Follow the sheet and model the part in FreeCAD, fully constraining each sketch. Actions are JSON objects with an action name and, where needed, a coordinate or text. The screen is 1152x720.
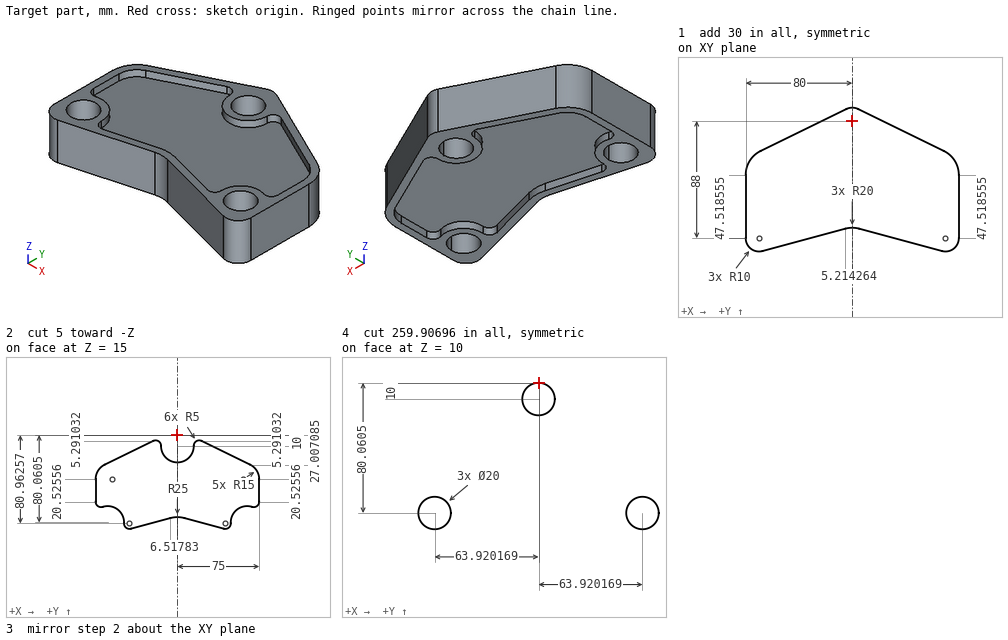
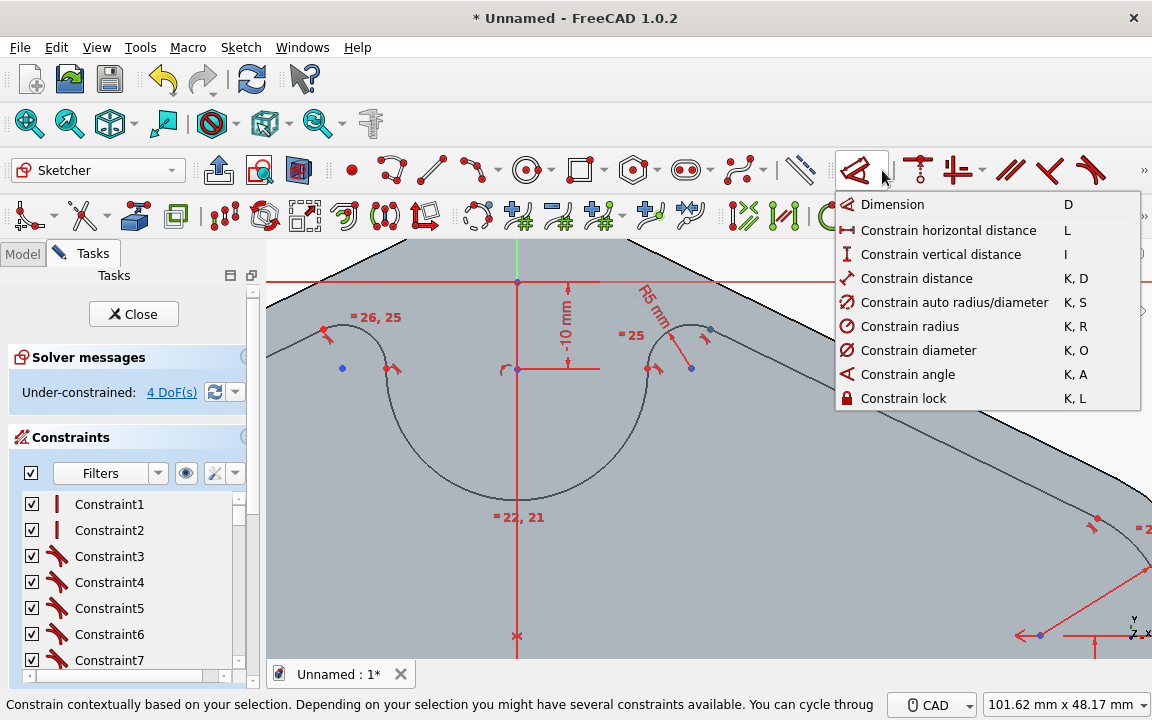
{"action": "left_click", "coordinate": [988, 254]}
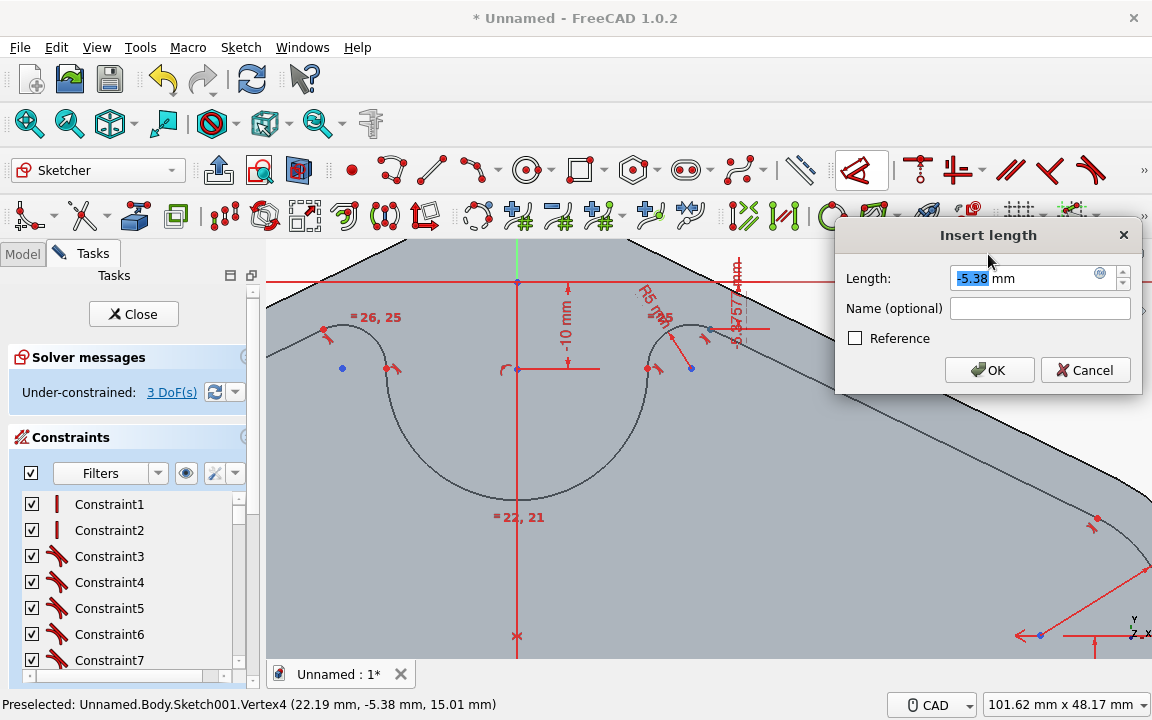
{"action": "type", "text": "-5.291032"}
{"action": "key", "text": "Return"}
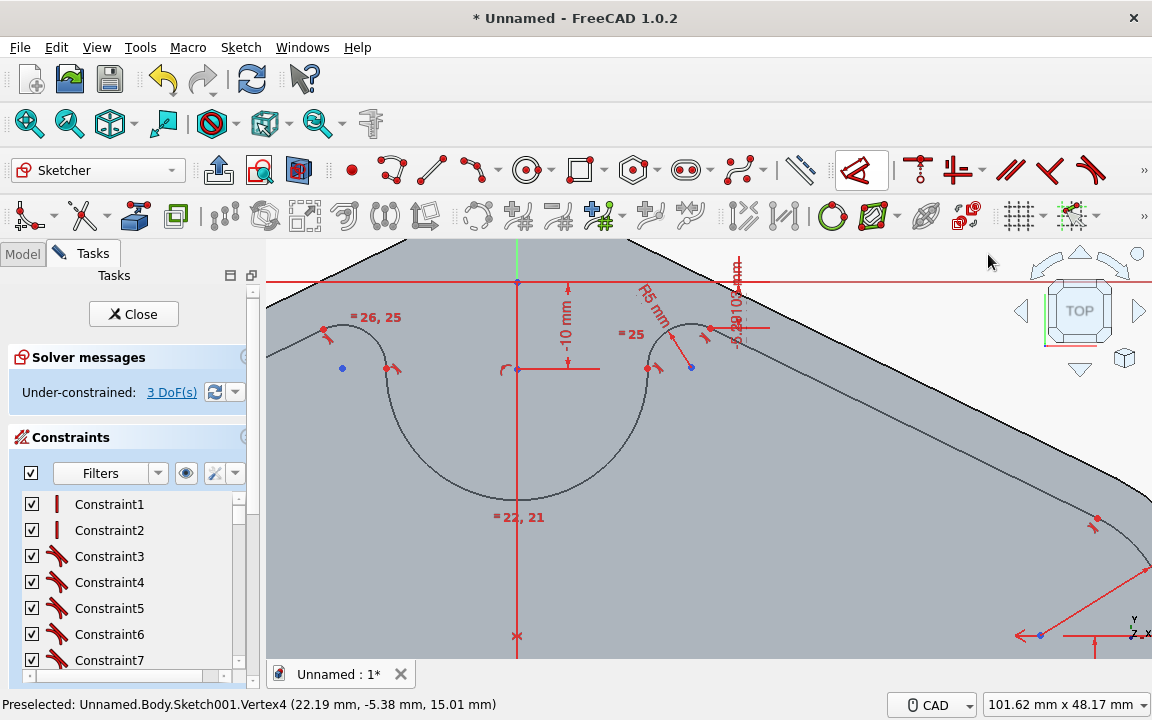
{"action": "left_click", "coordinate": [324, 329]}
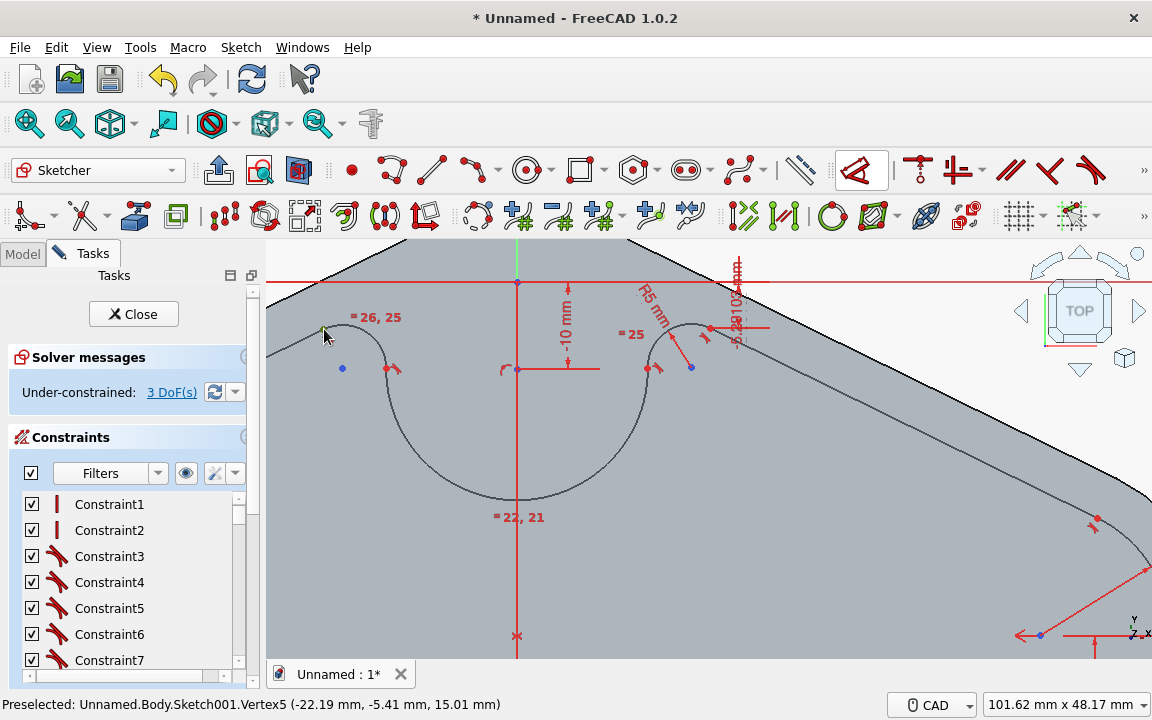
{"action": "key", "text": "i"}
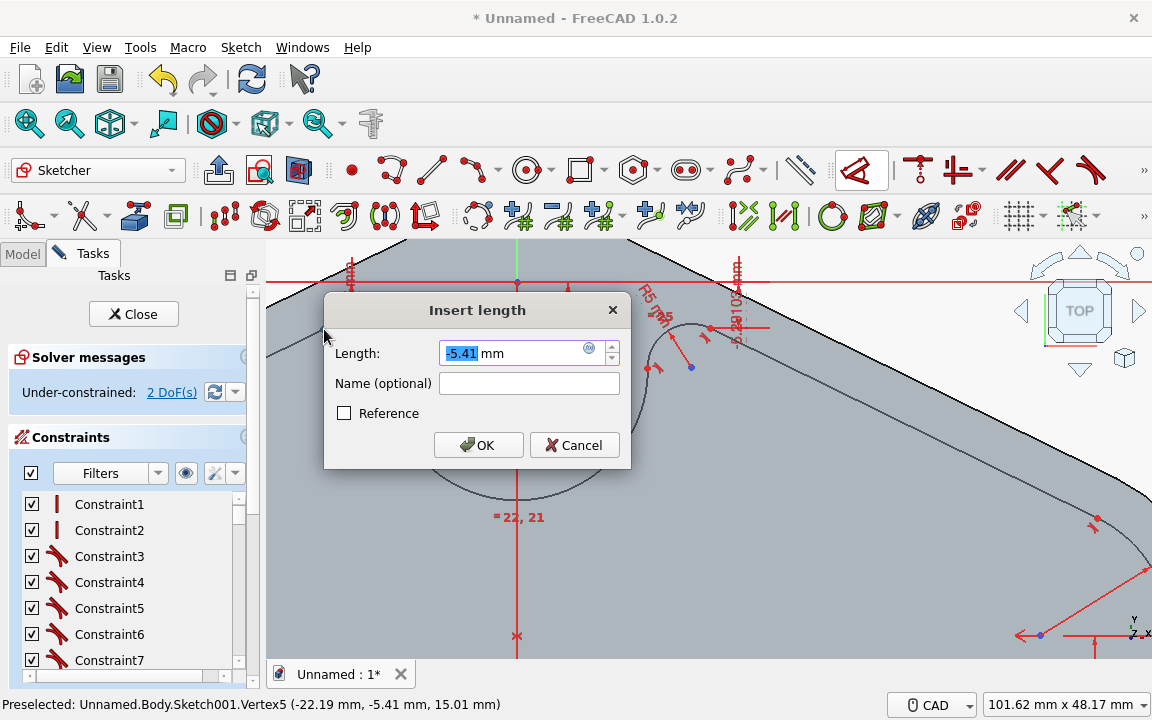
{"action": "type", "text": "-5.291032"}
{"action": "key", "text": "Return"}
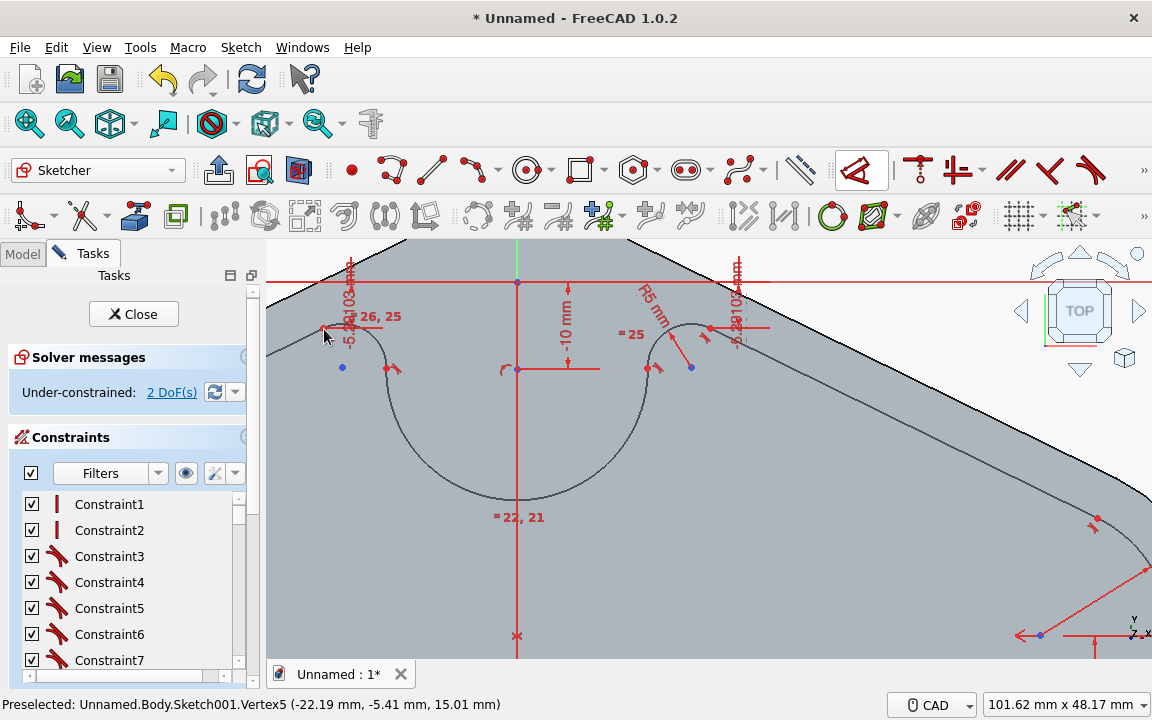
{"action": "scroll", "coordinate": [712, 328], "scroll_direction": "down", "scroll_amount": 5}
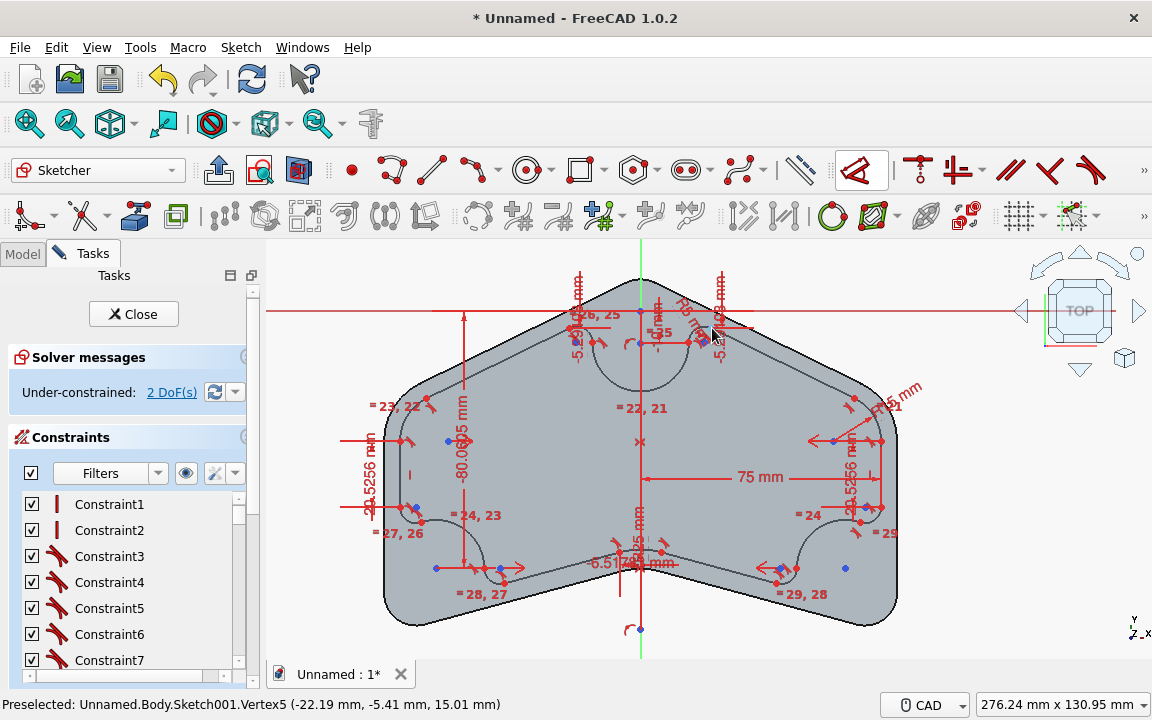
{"action": "left_click", "coordinate": [500, 568]}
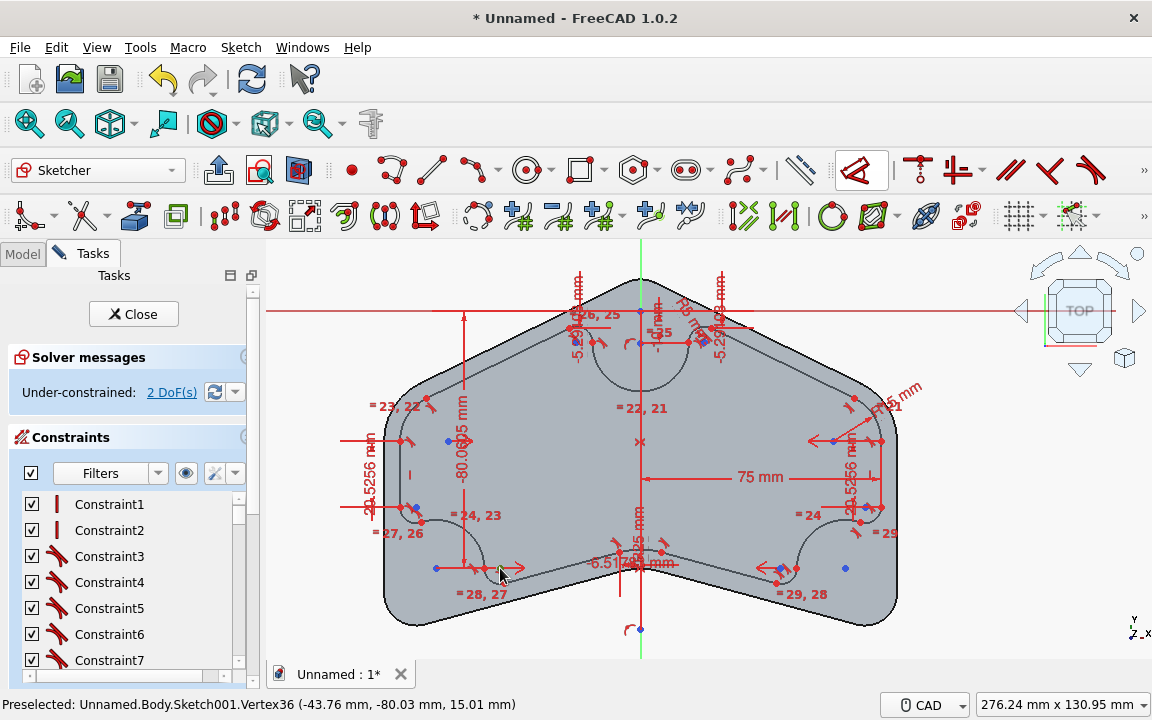
{"action": "key", "text": "i"}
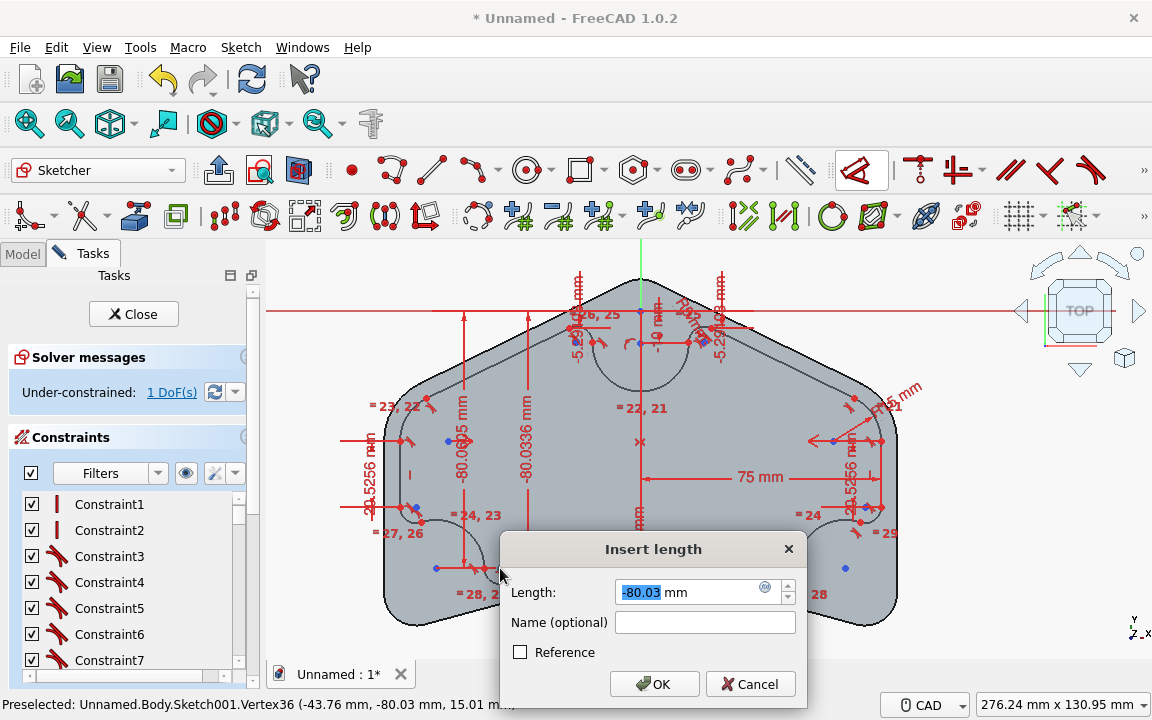
{"action": "type", "text": "-80.96257"}
{"action": "key", "text": "Return"}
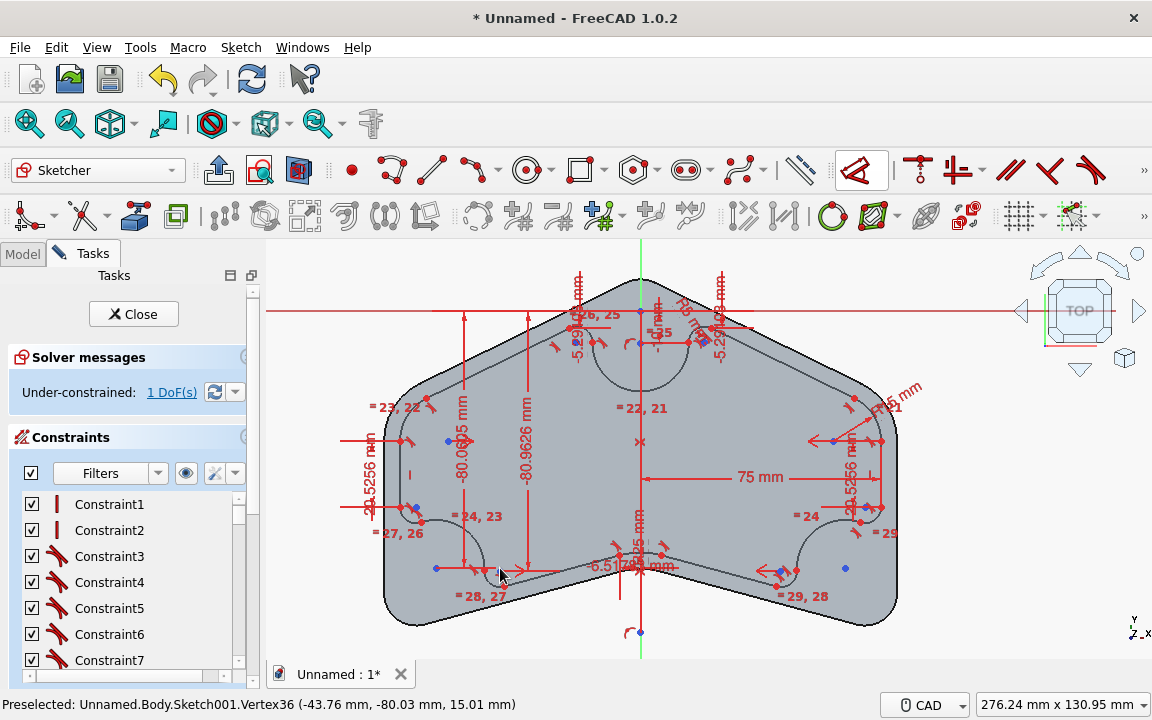
{"action": "left_click", "coordinate": [854, 398]}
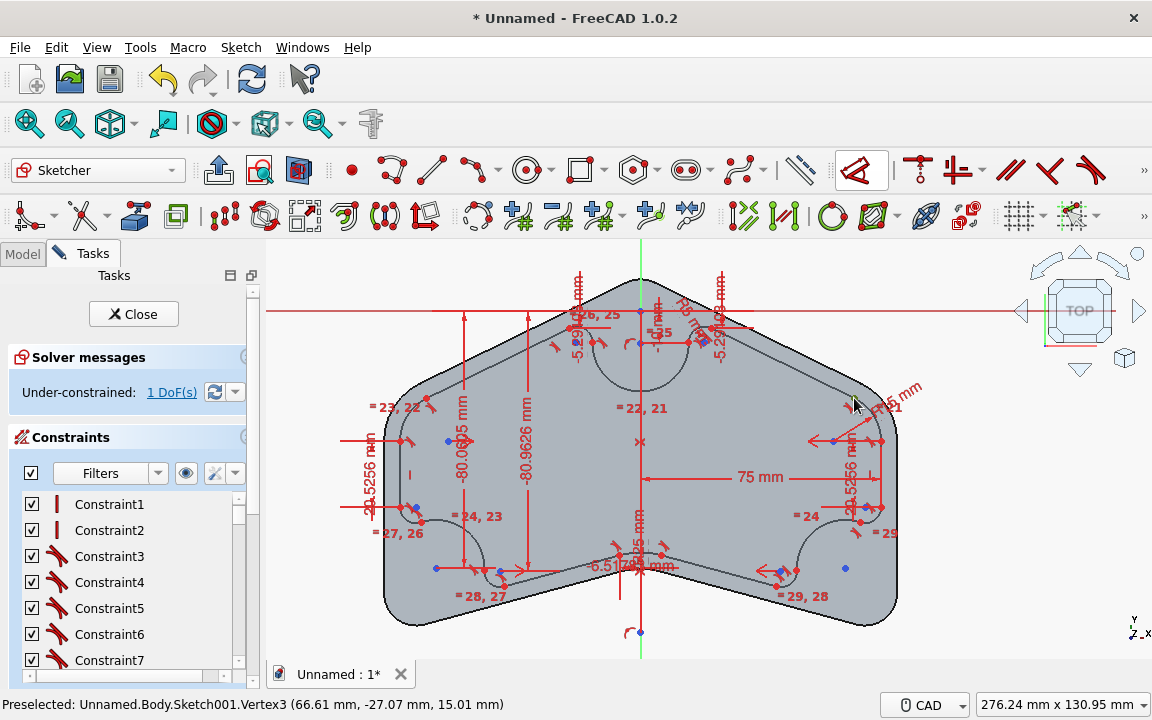
{"action": "key", "text": "i"}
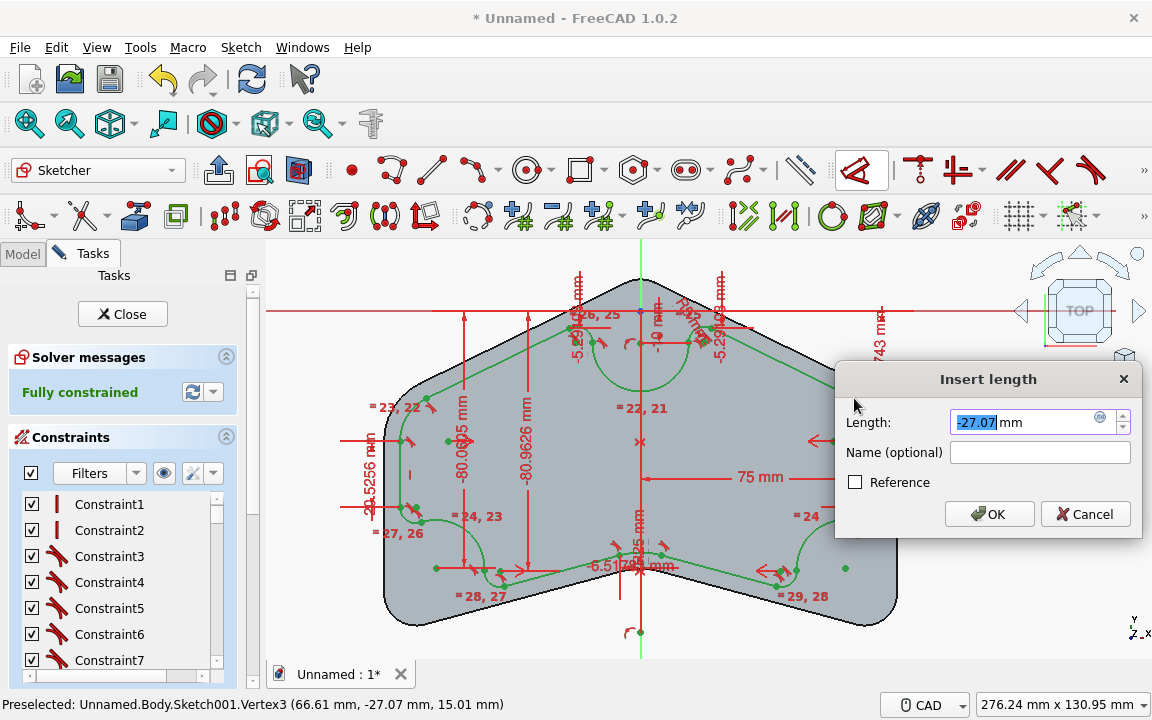
{"action": "type", "text": "-27.007085"}
{"action": "key", "text": "Return"}